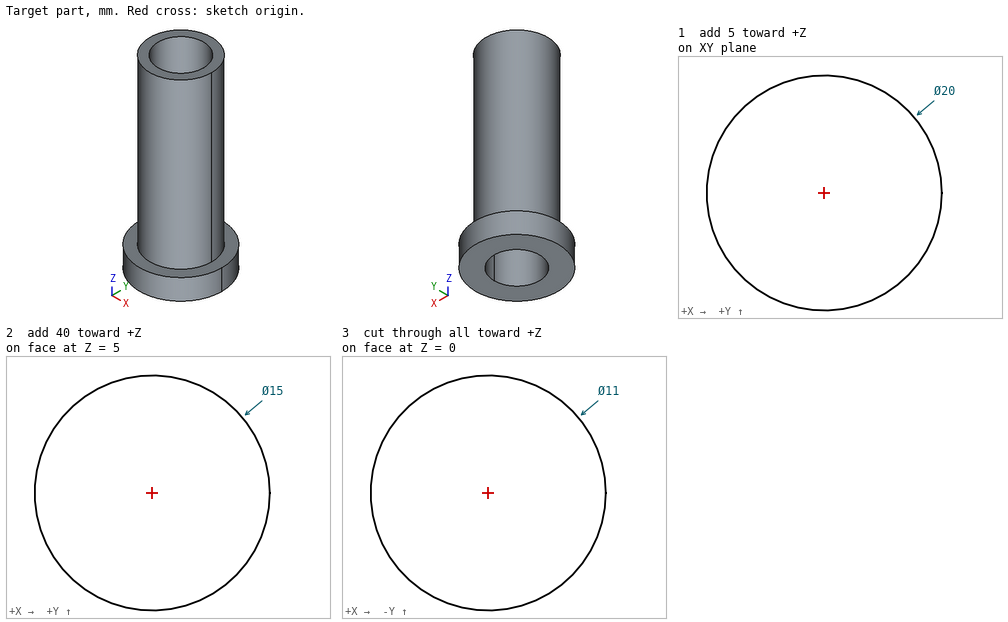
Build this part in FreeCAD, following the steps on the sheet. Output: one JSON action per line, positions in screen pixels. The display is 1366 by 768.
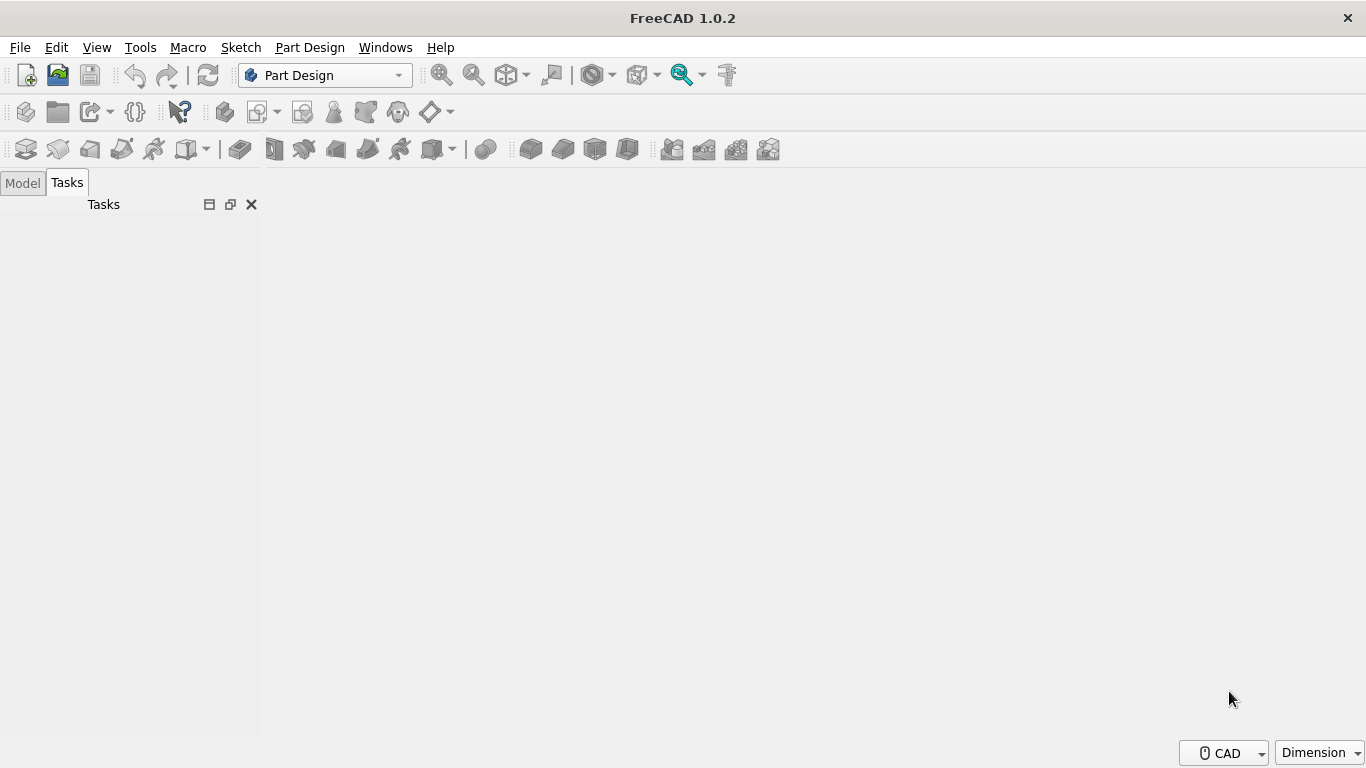
{"action": "key", "text": "ctrl+n"}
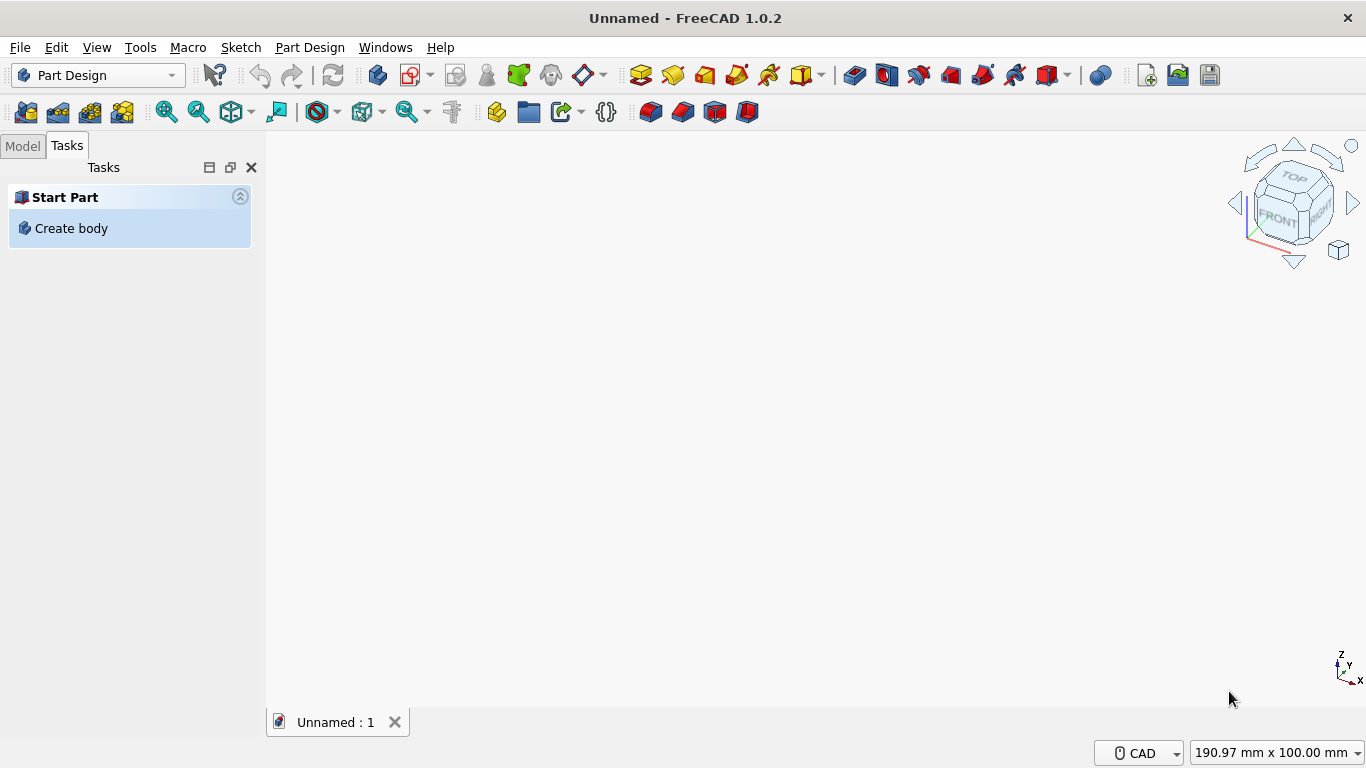
{"action": "left_click", "coordinate": [410, 76]}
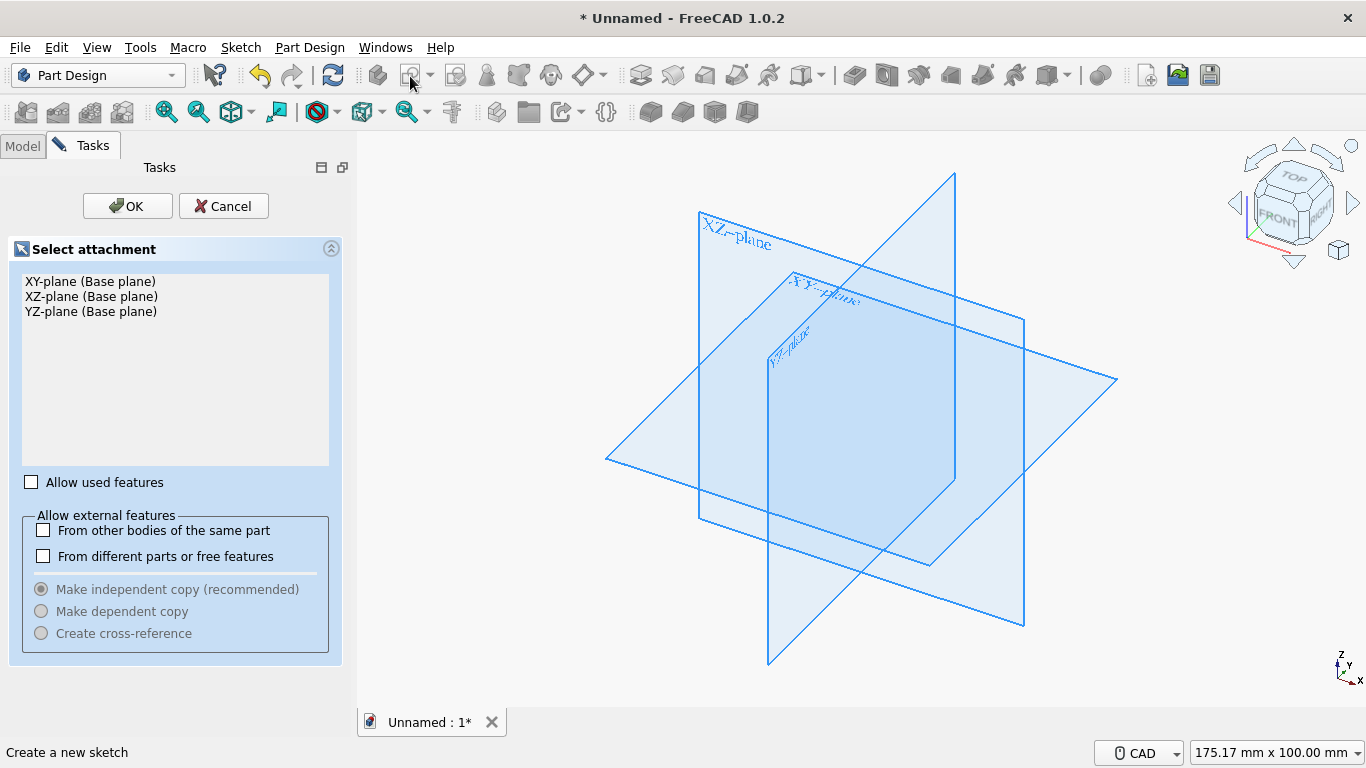
{"action": "left_click", "coordinate": [82, 282]}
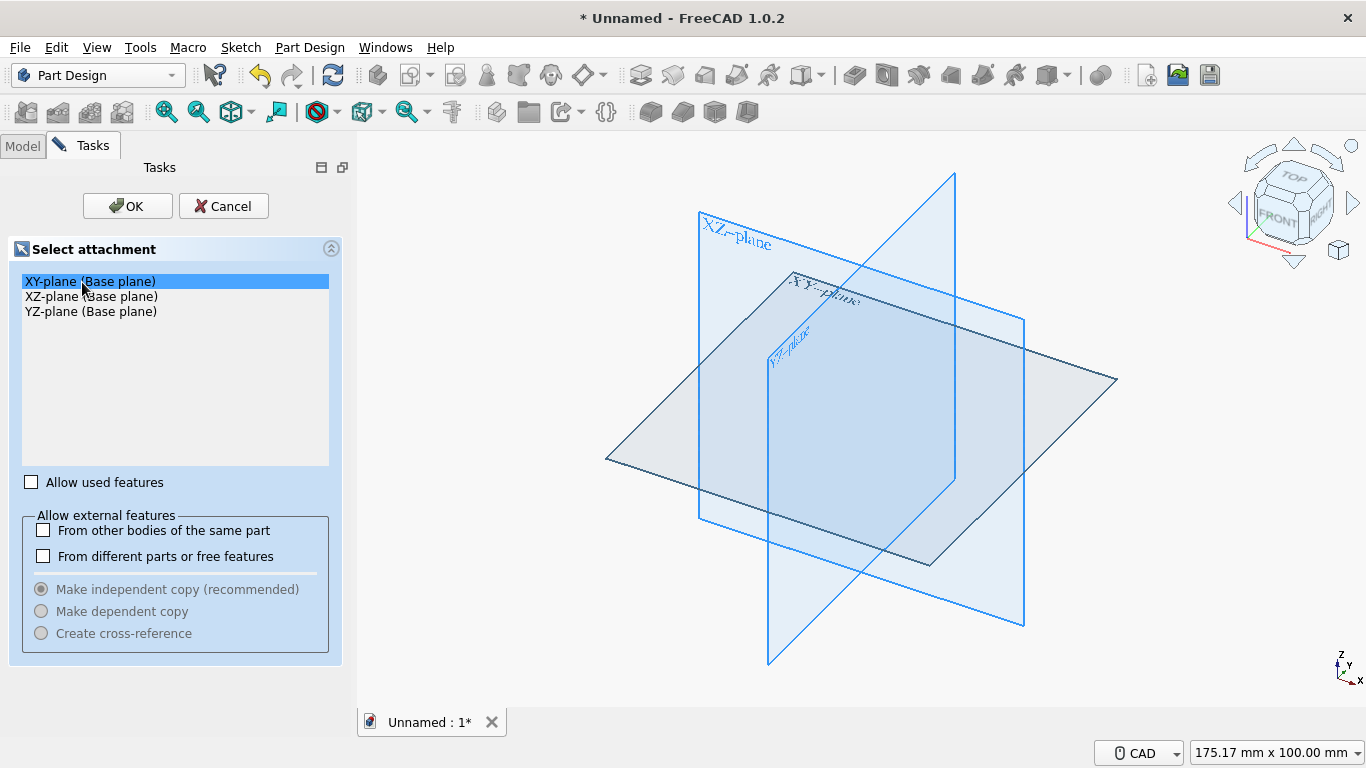
{"action": "left_click", "coordinate": [128, 206]}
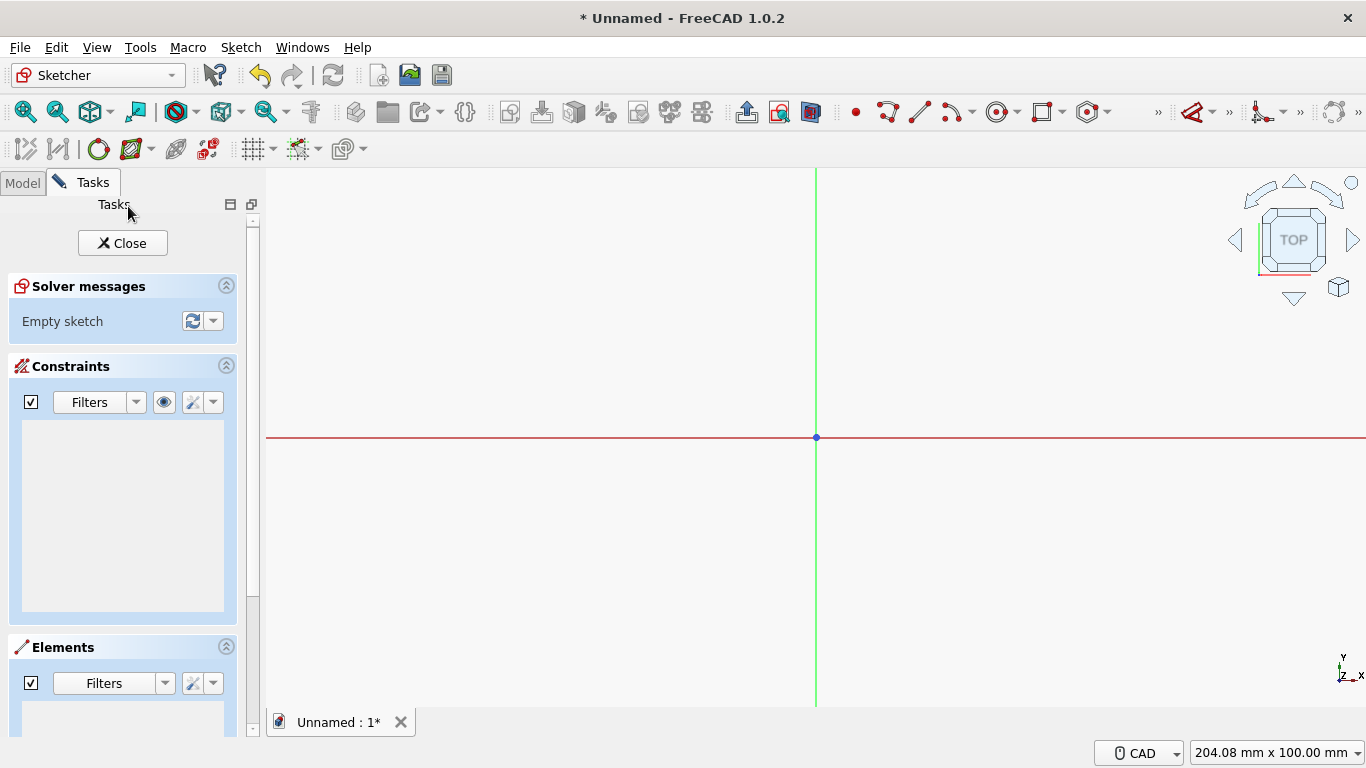
{"action": "scroll", "coordinate": [846, 438], "scroll_direction": "up", "scroll_amount": 6}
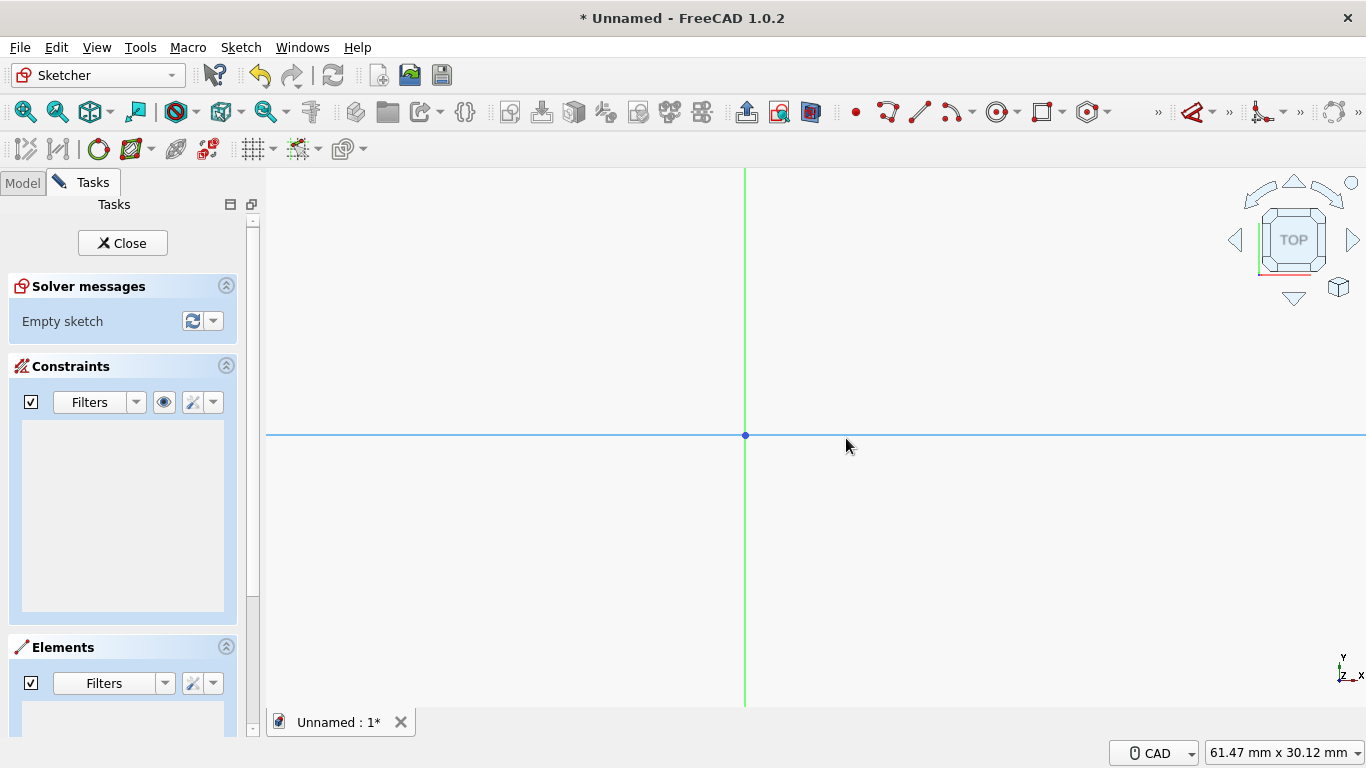
{"action": "key", "text": "g c"}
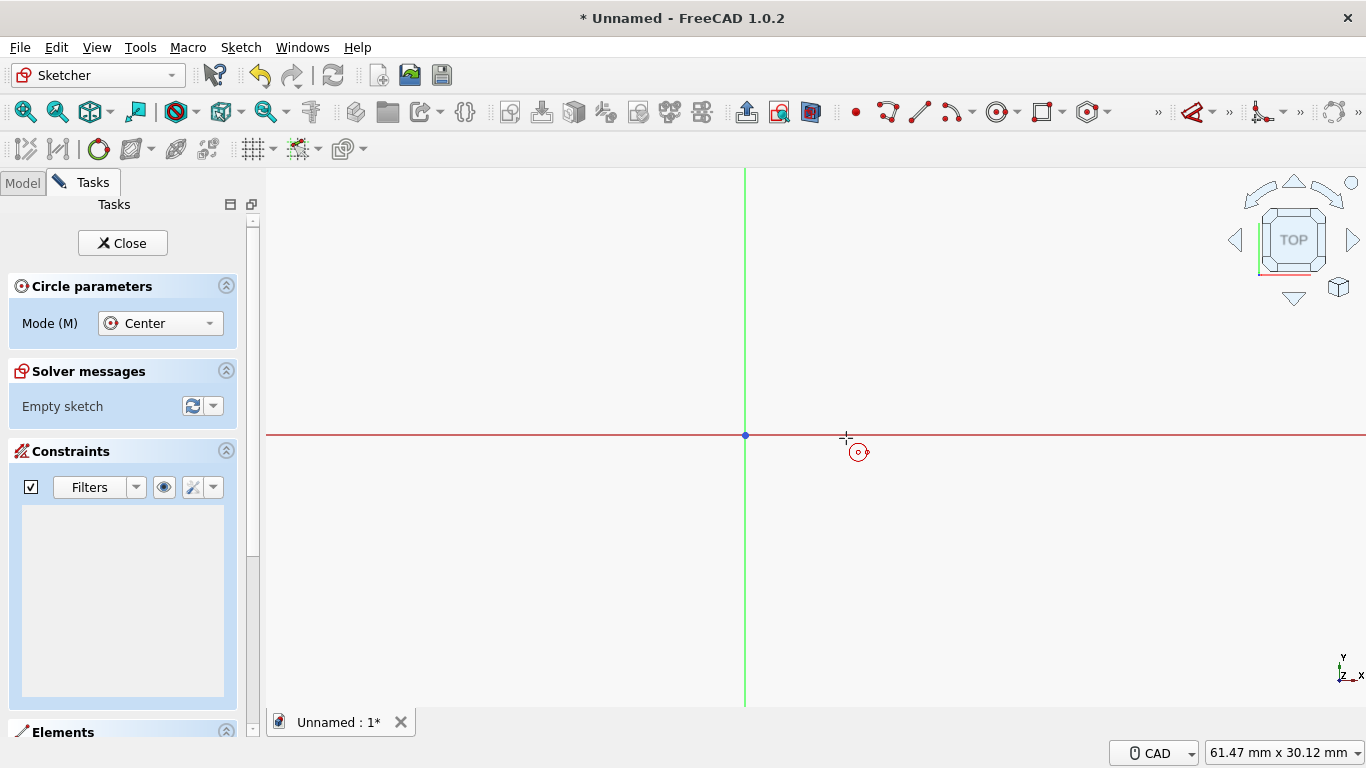
{"action": "left_click", "coordinate": [745, 435]}
{"action": "mouse_move", "coordinate": [872, 309]}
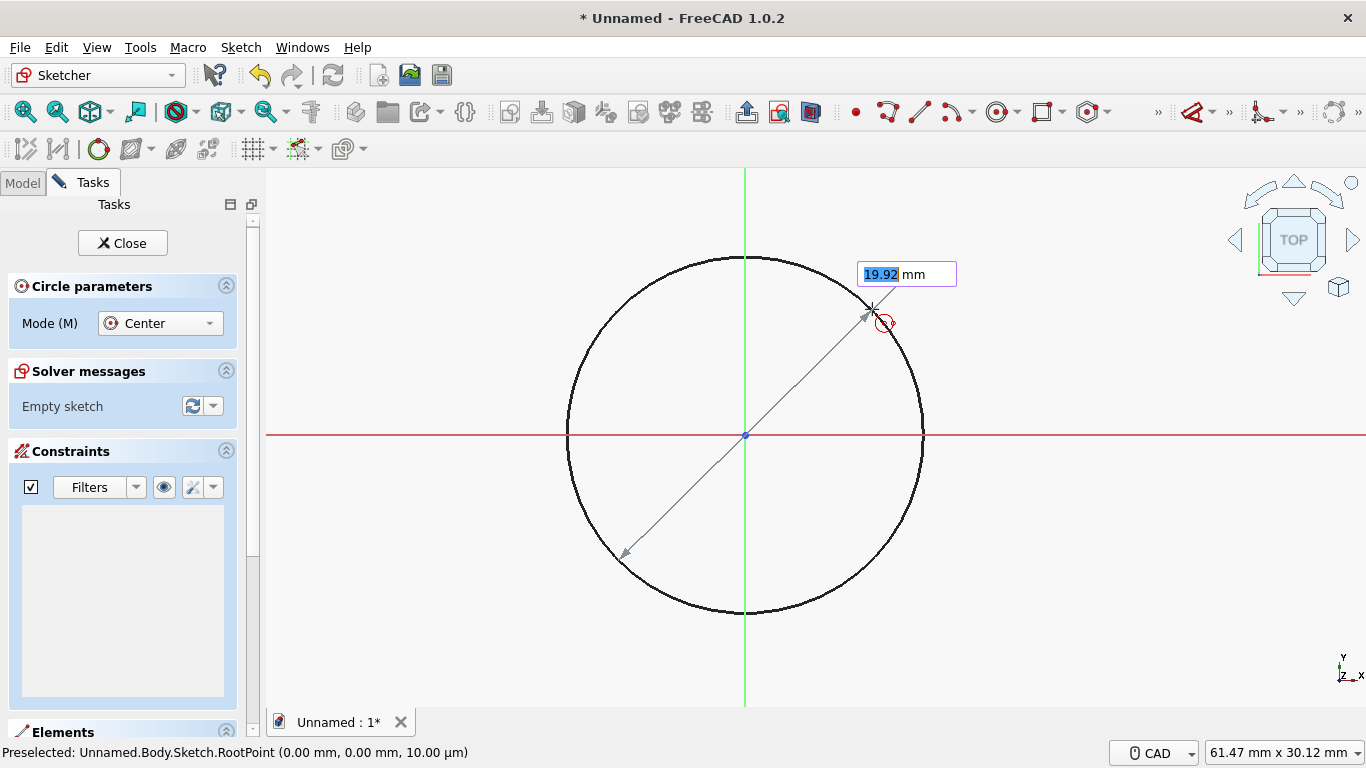
{"action": "type", "text": "20"}
{"action": "key", "text": "Return"}
{"action": "key", "text": "Escape"}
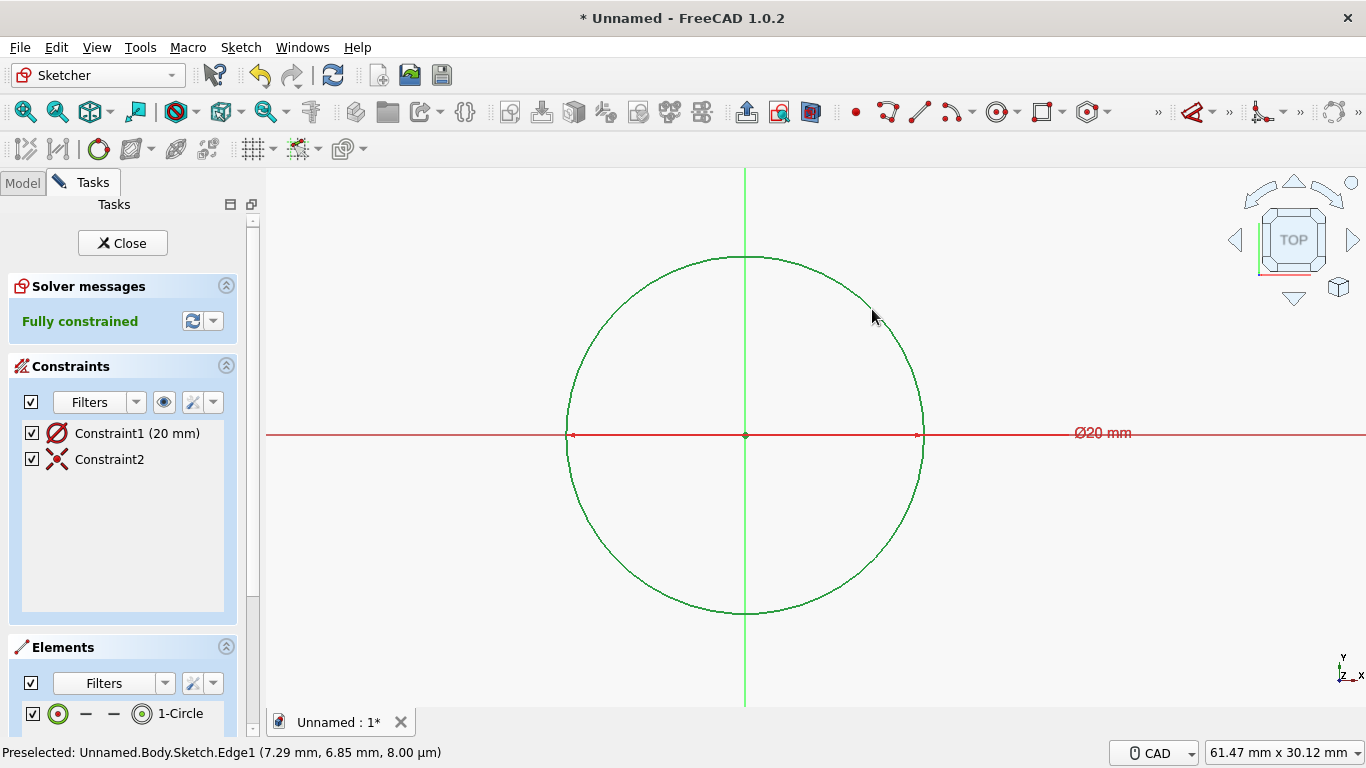
{"action": "left_click", "coordinate": [123, 243]}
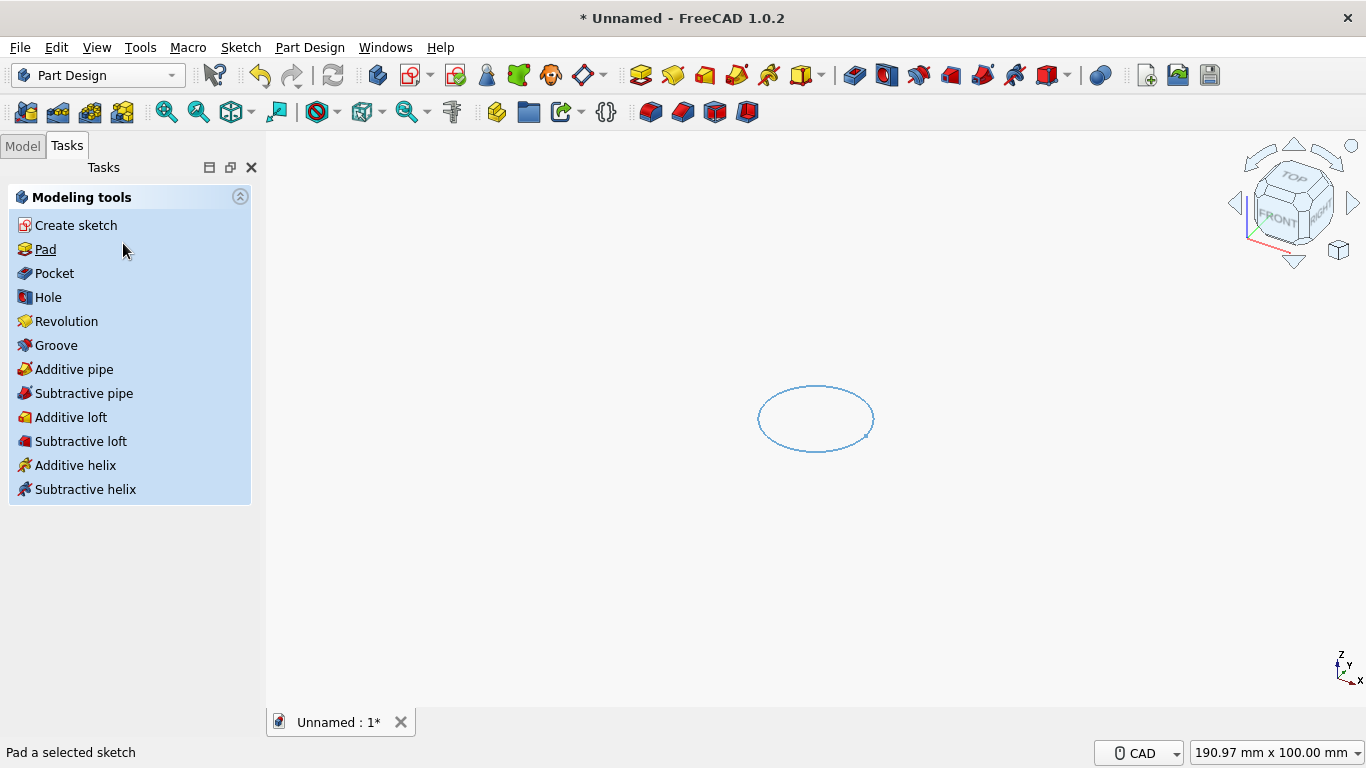
{"action": "left_click", "coordinate": [642, 76]}